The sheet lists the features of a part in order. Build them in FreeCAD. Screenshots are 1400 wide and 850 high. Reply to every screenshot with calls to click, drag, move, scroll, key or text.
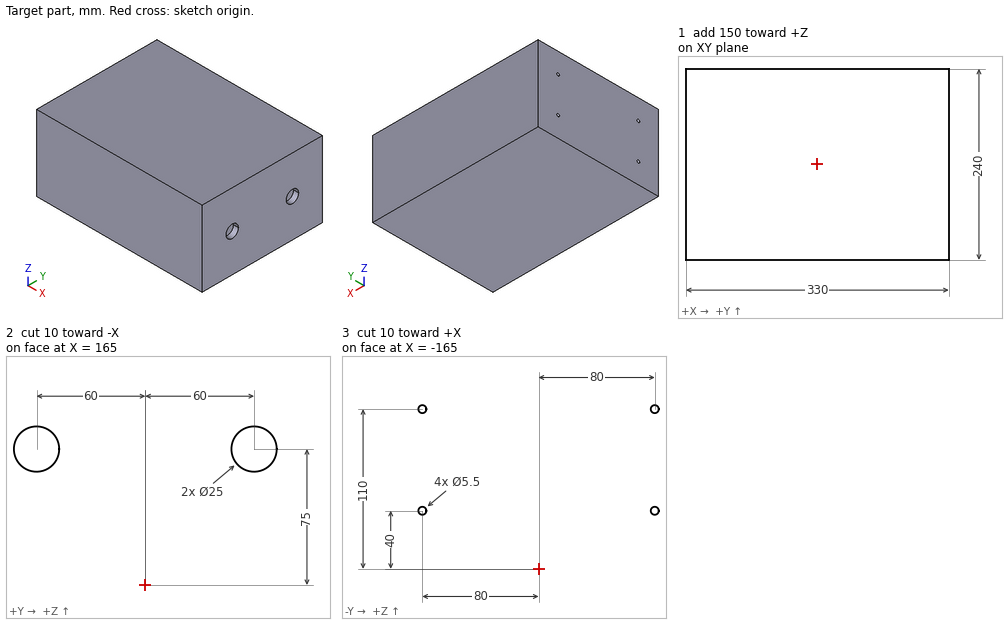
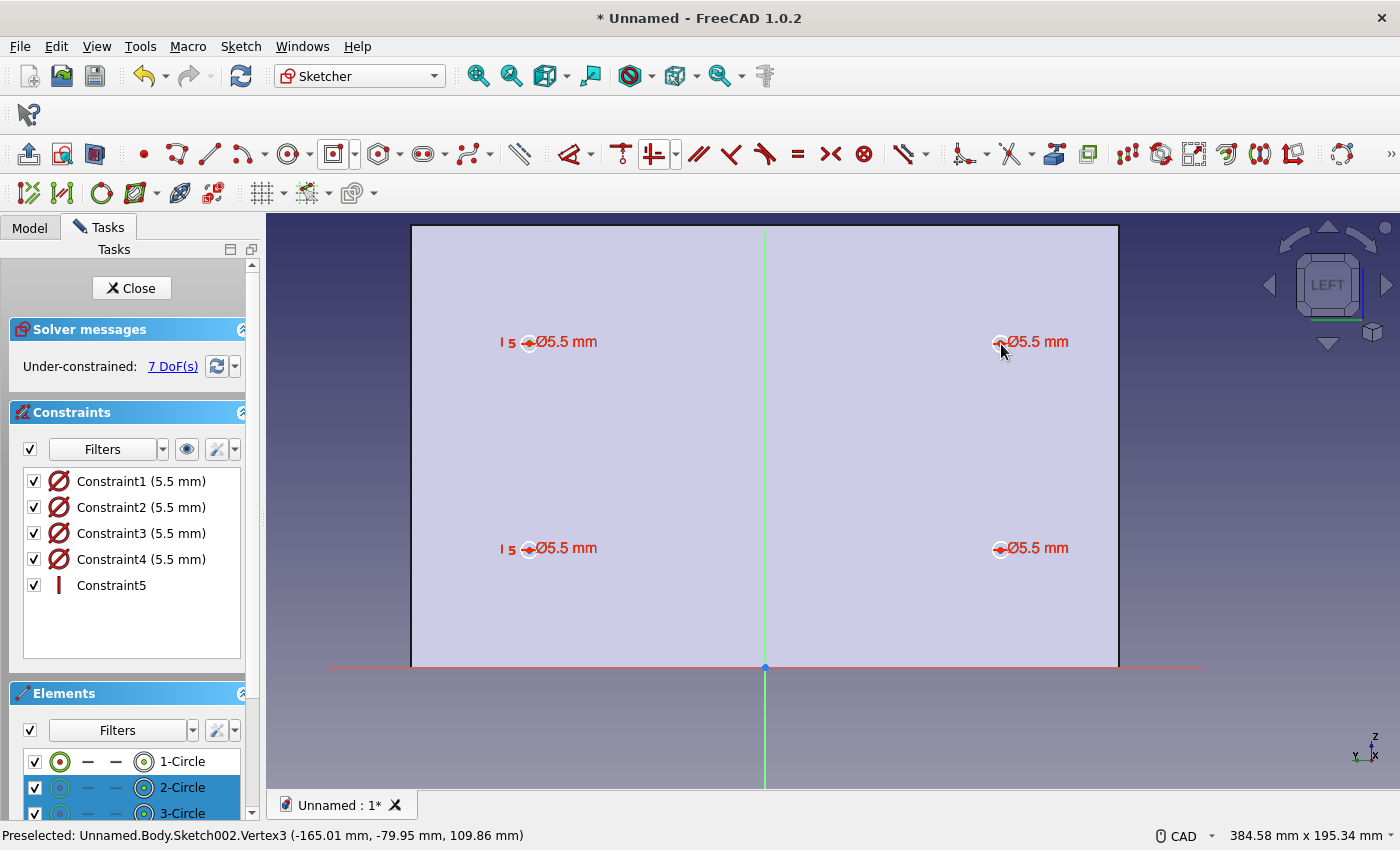
key(h)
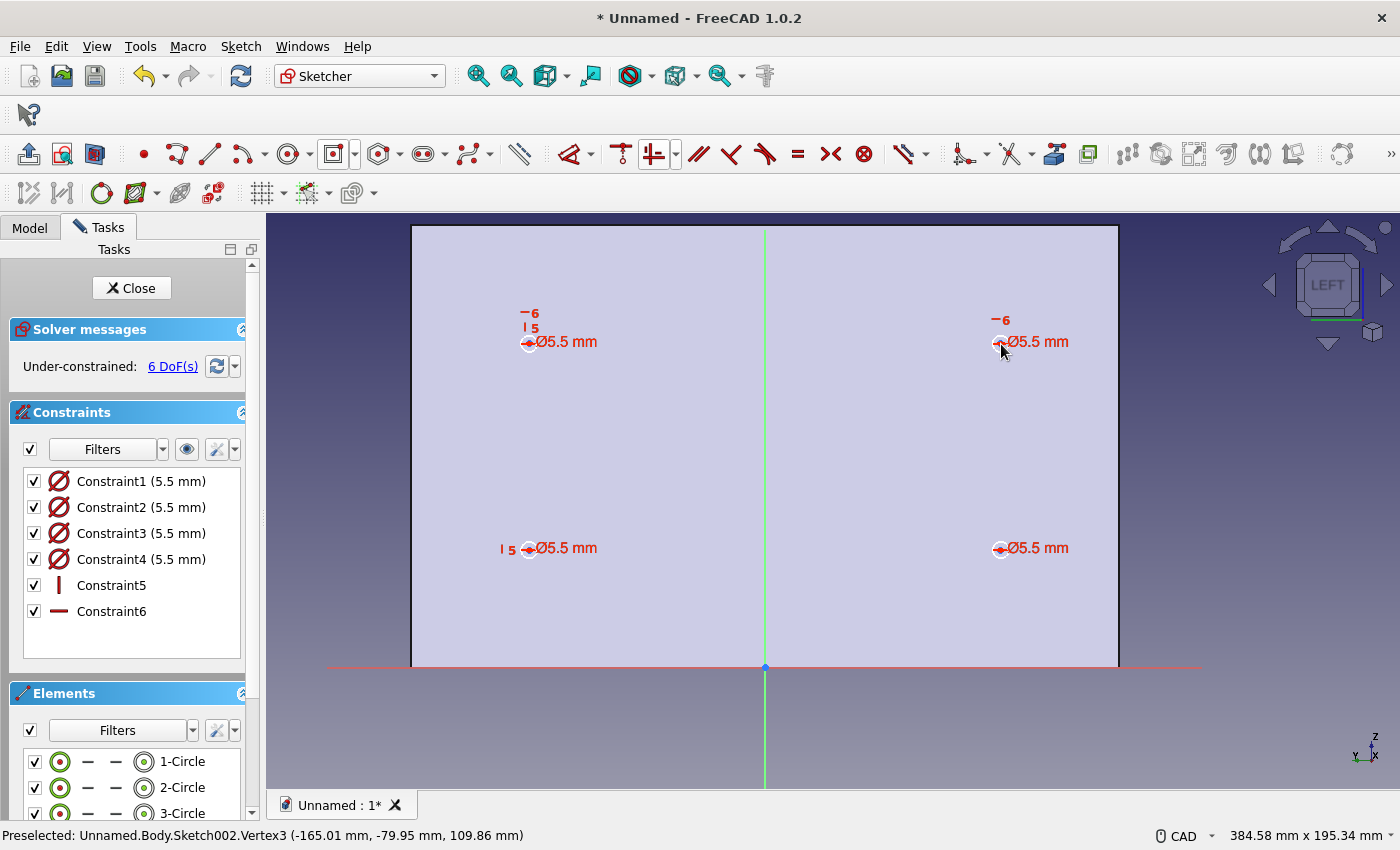
click(1001, 344)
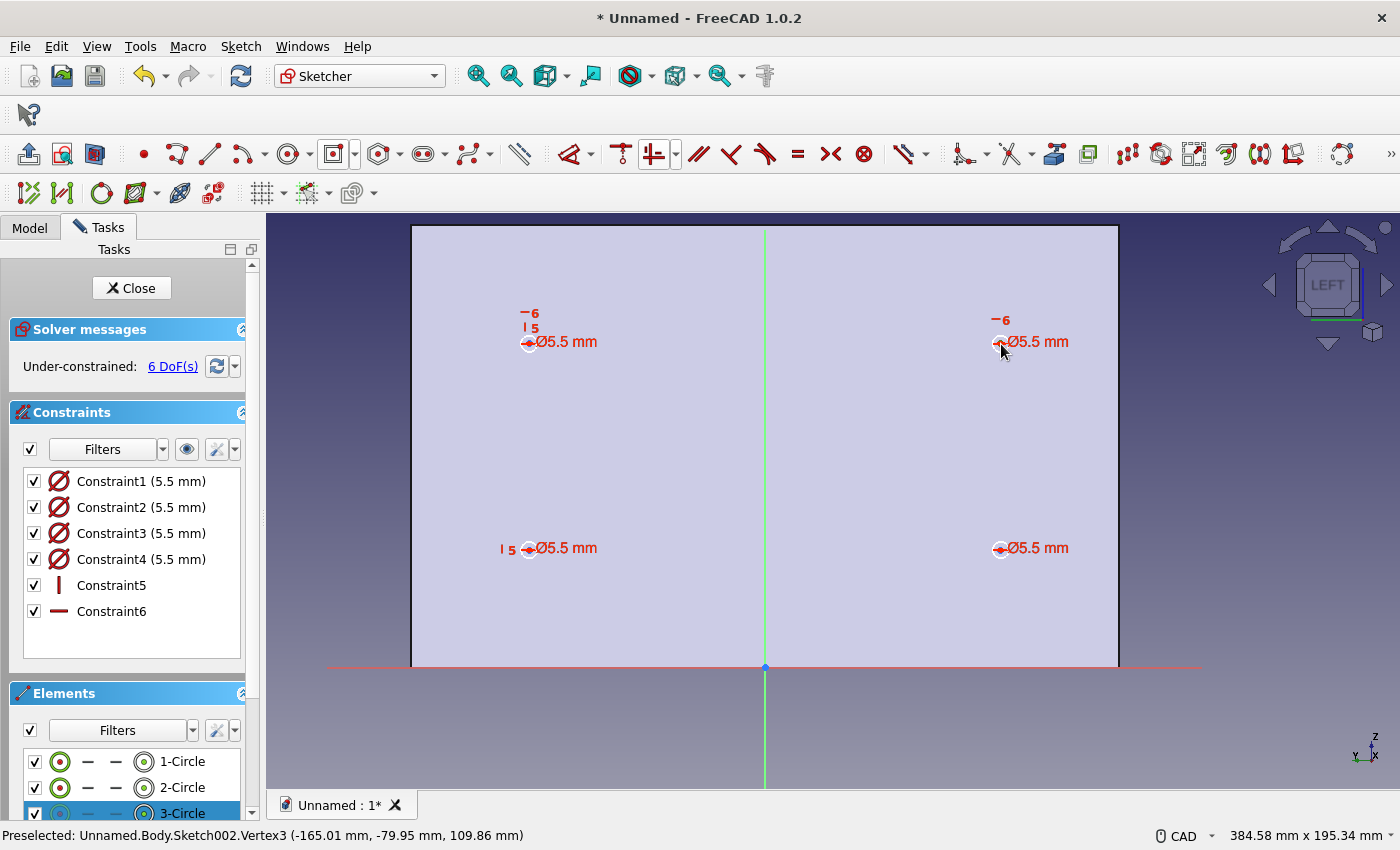
click(1001, 550)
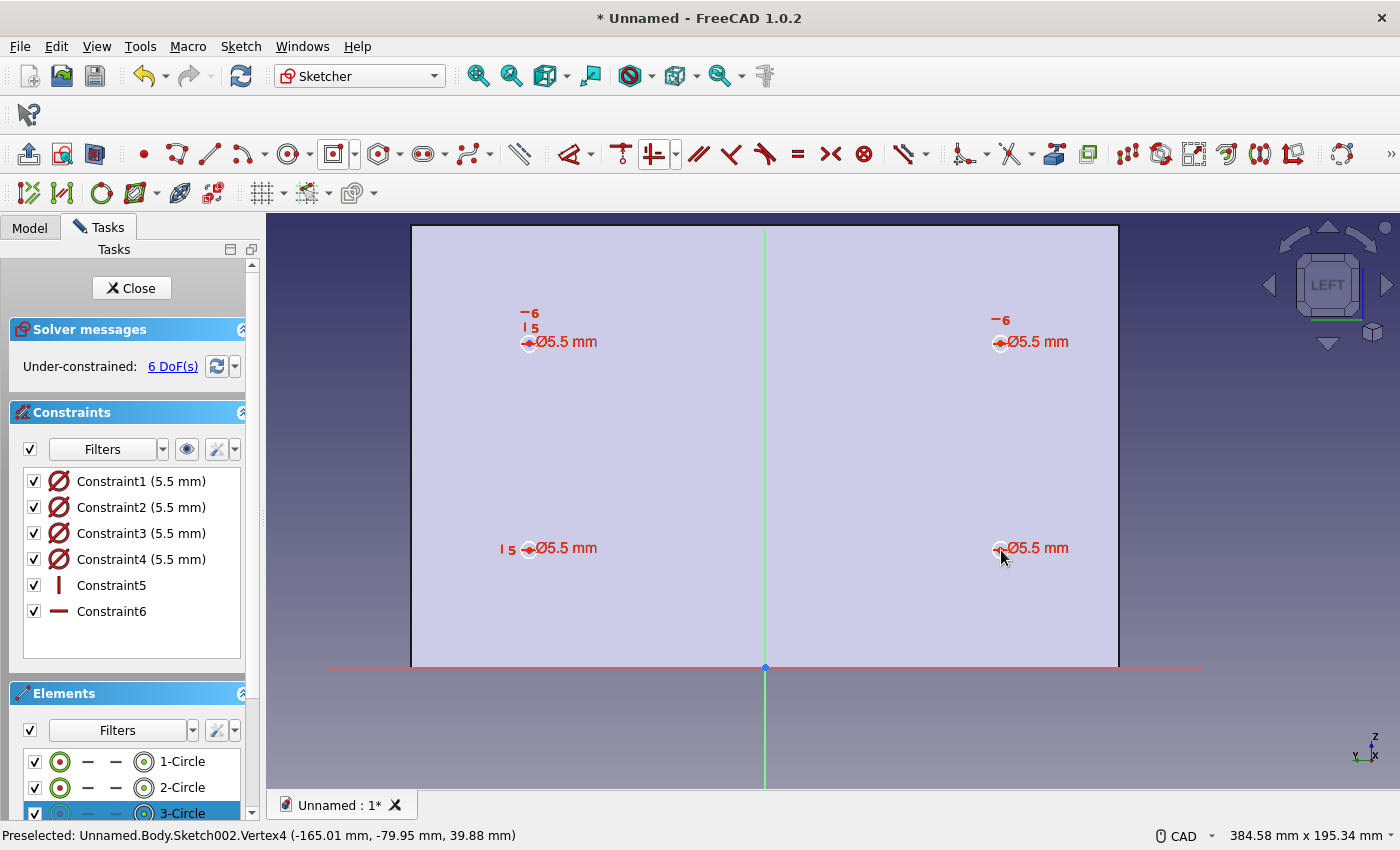
key(v)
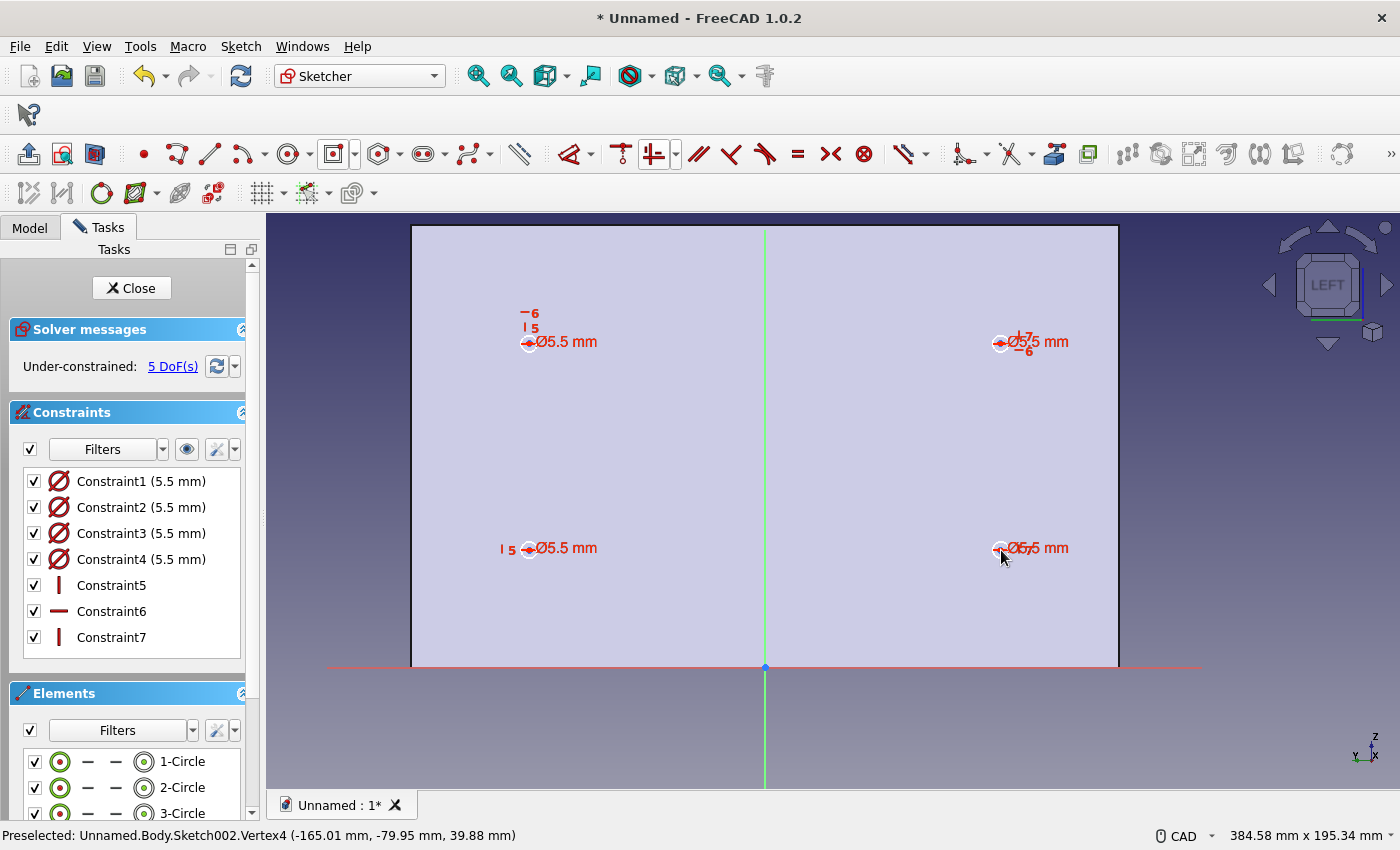
click(529, 550)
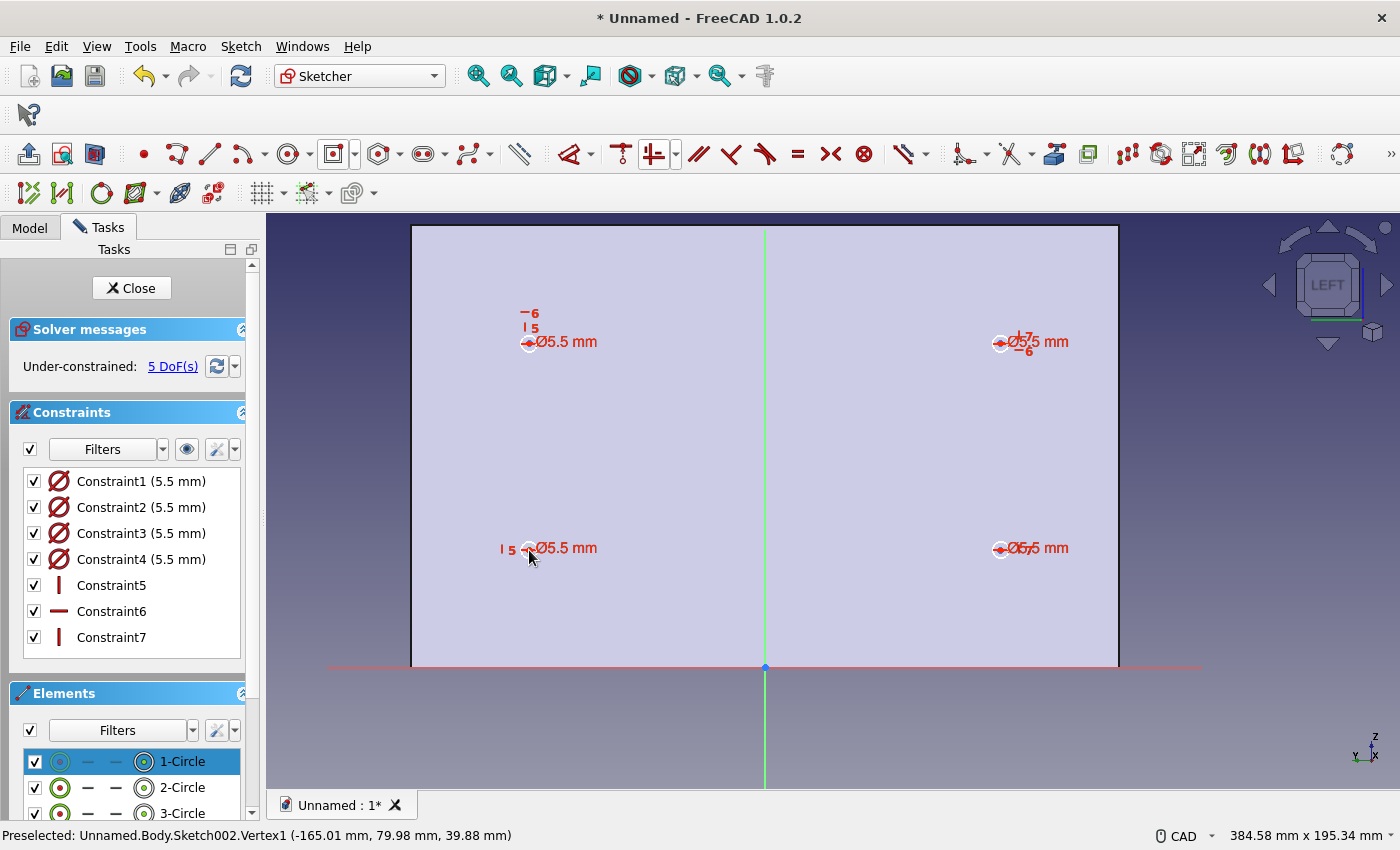
click(1001, 550)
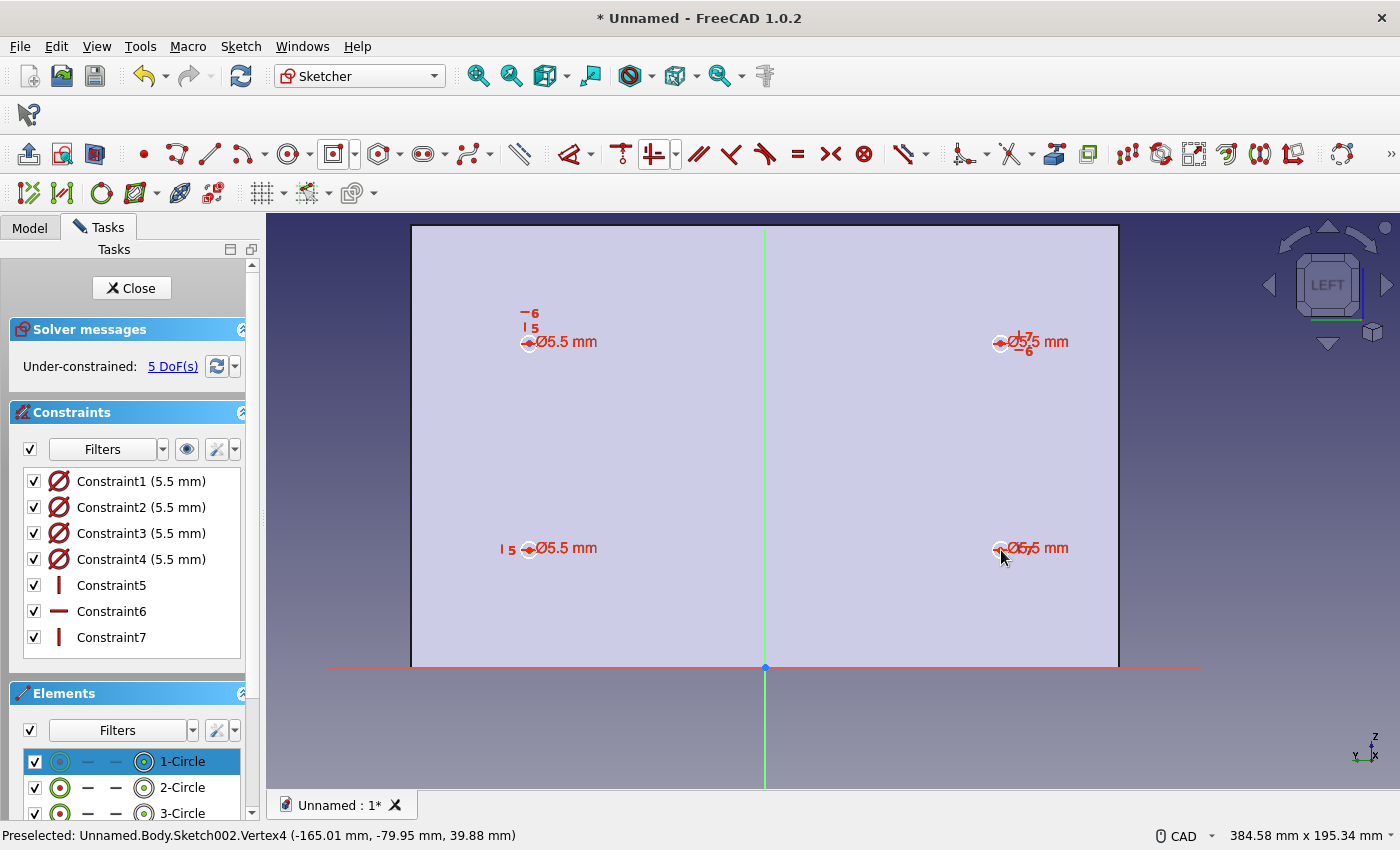
key(h)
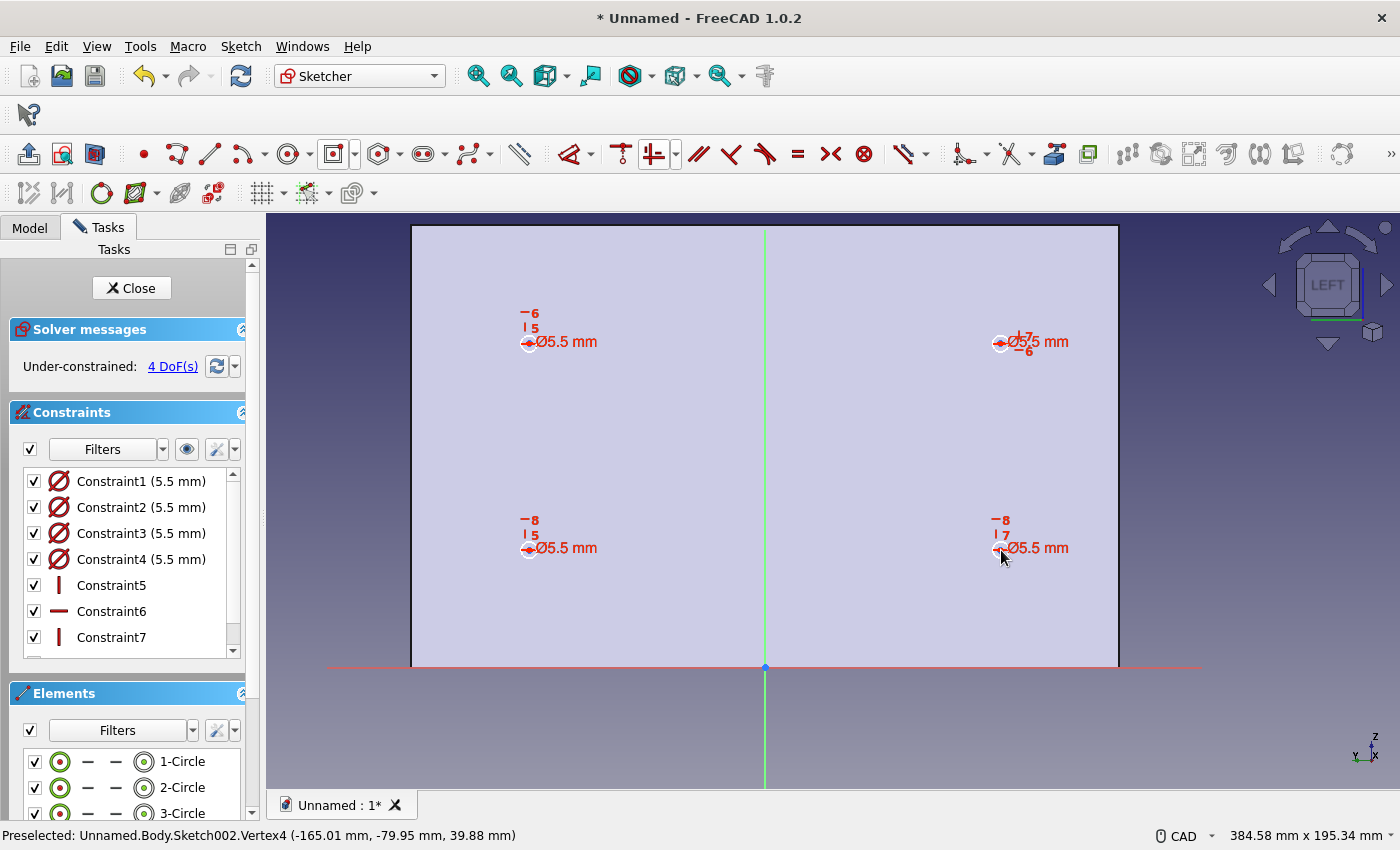
click(568, 154)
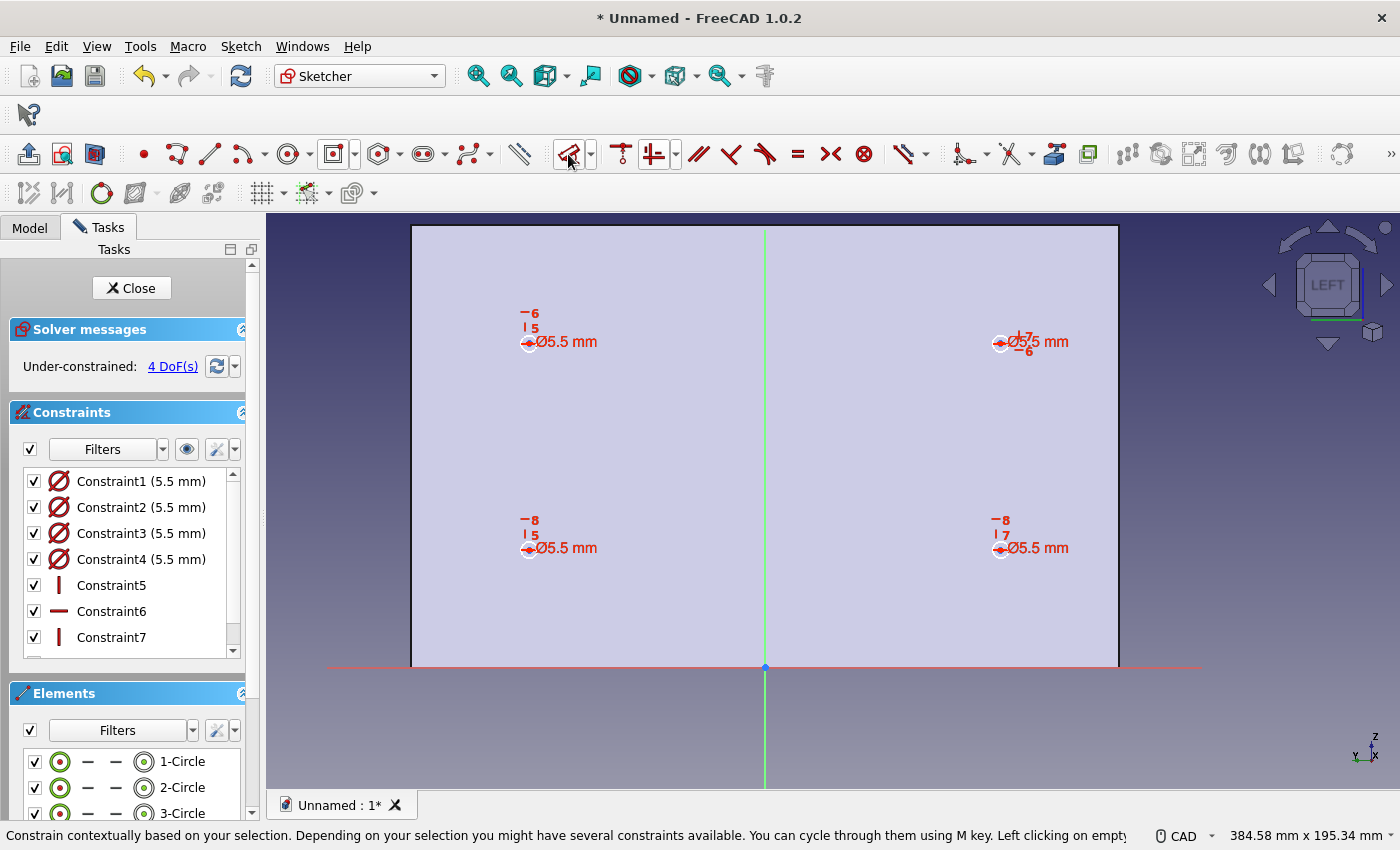
click(529, 550)
click(647, 702)